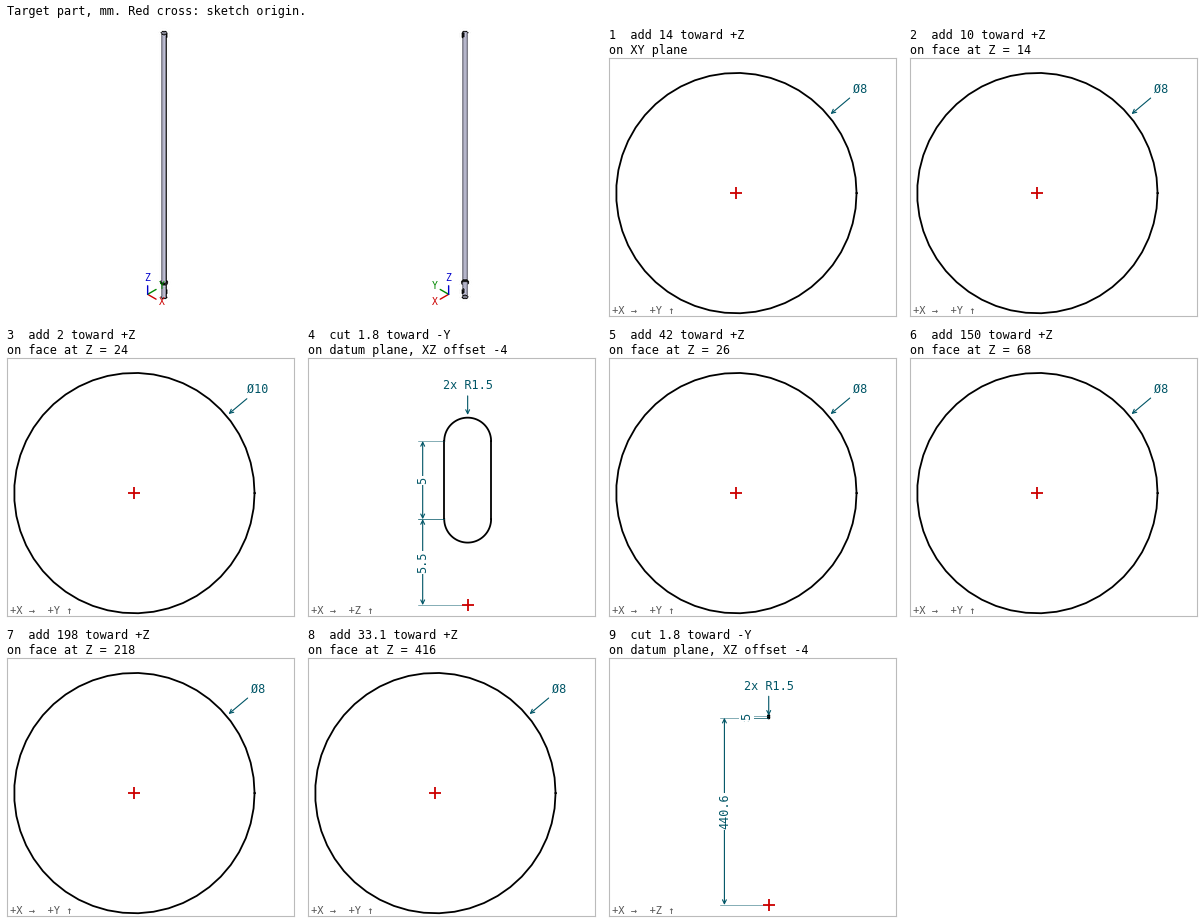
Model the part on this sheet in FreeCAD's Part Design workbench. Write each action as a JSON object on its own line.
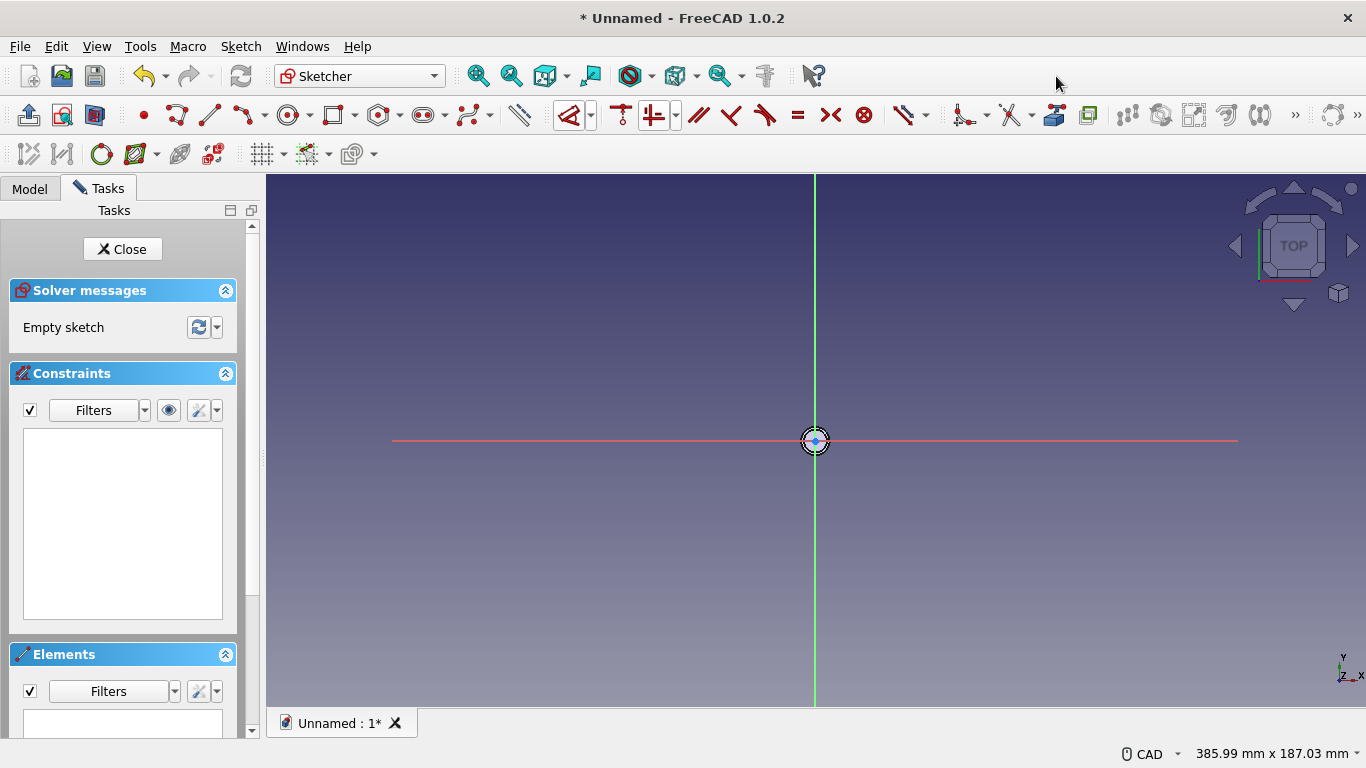
{"action": "scroll", "coordinate": [821, 441], "scroll_direction": "up", "scroll_amount": 13}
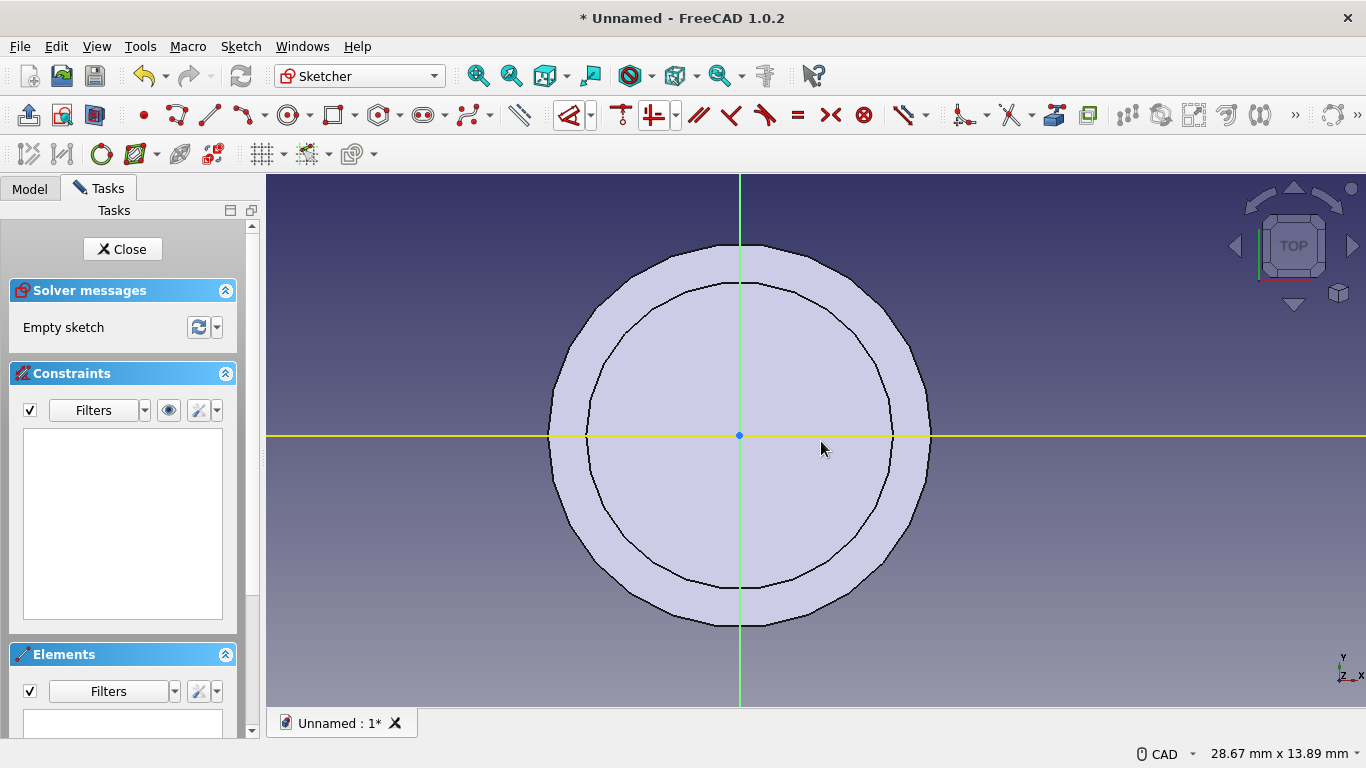
{"action": "left_click", "coordinate": [288, 116]}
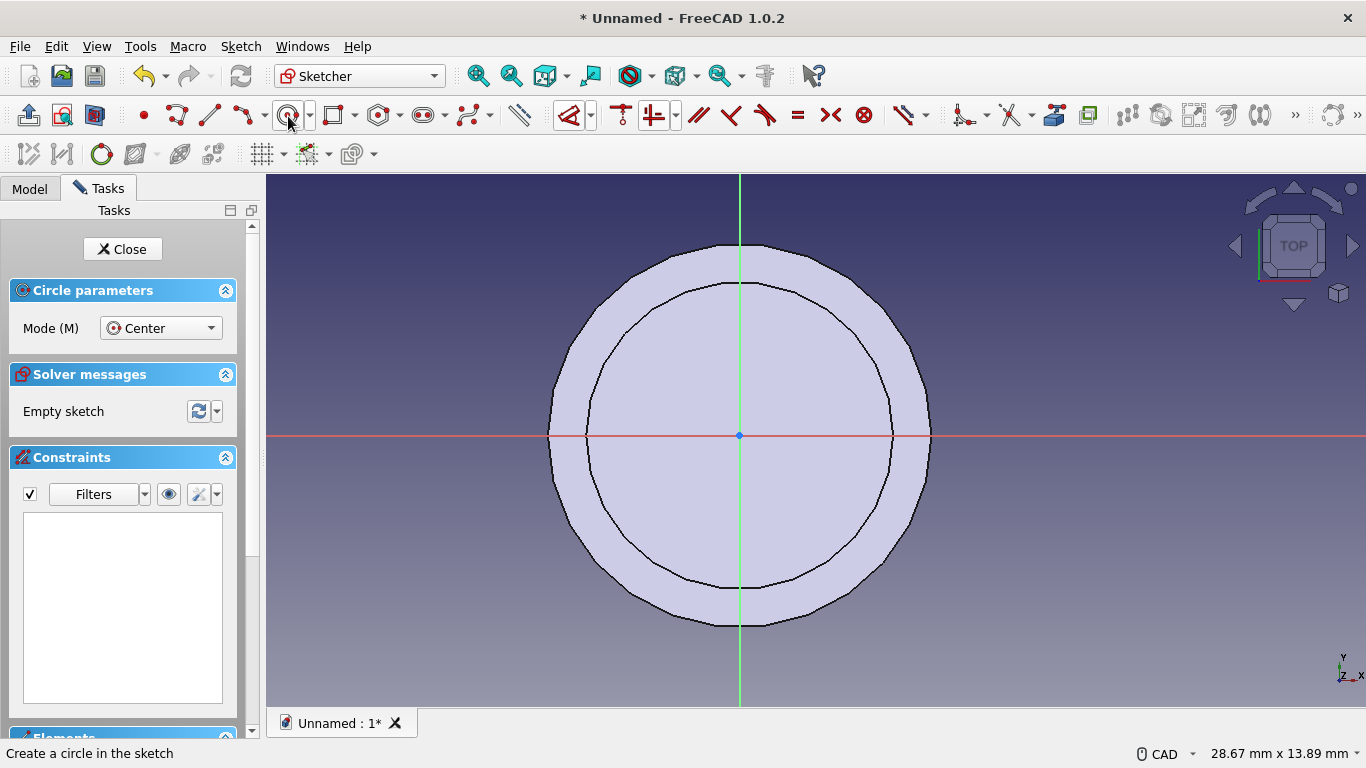
{"action": "left_click", "coordinate": [740, 436]}
{"action": "left_click", "coordinate": [848, 327]}
{"action": "key", "text": "Escape"}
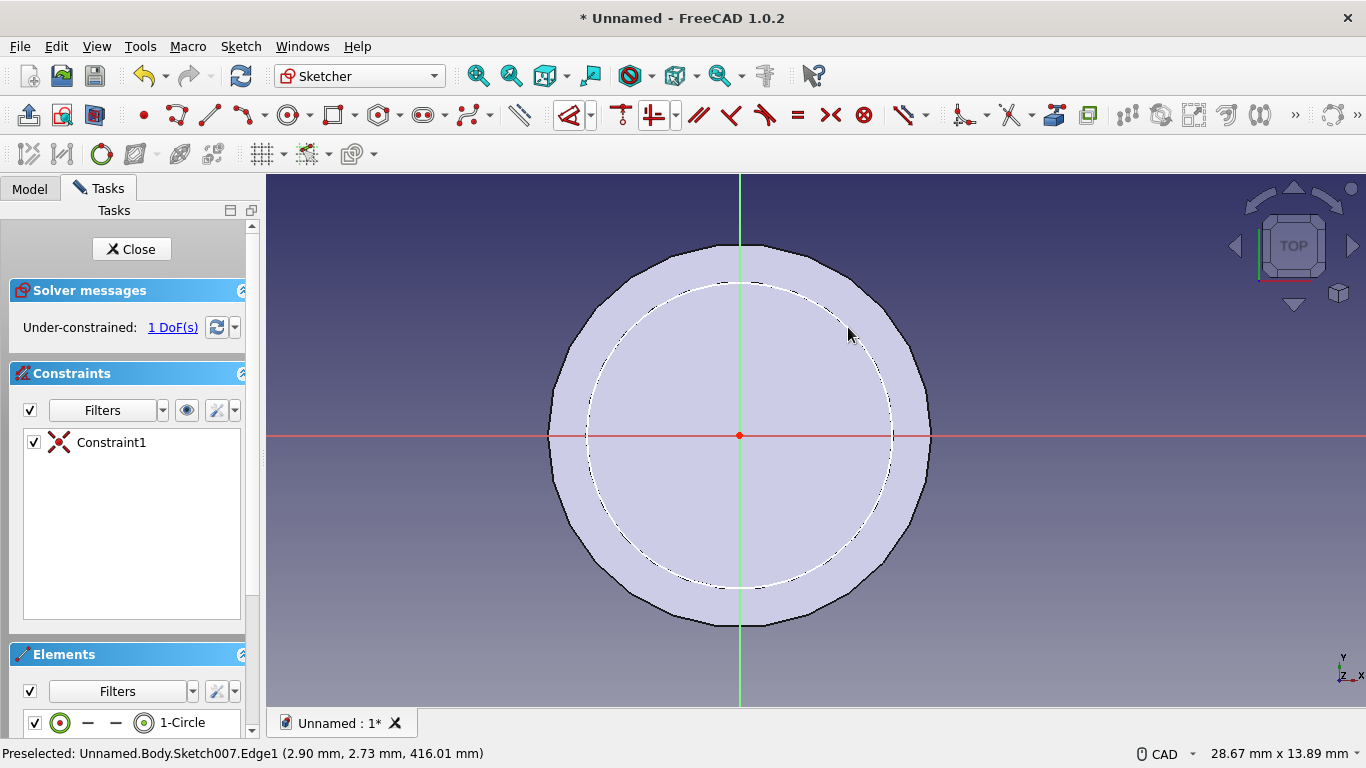
{"action": "left_click", "coordinate": [847, 327]}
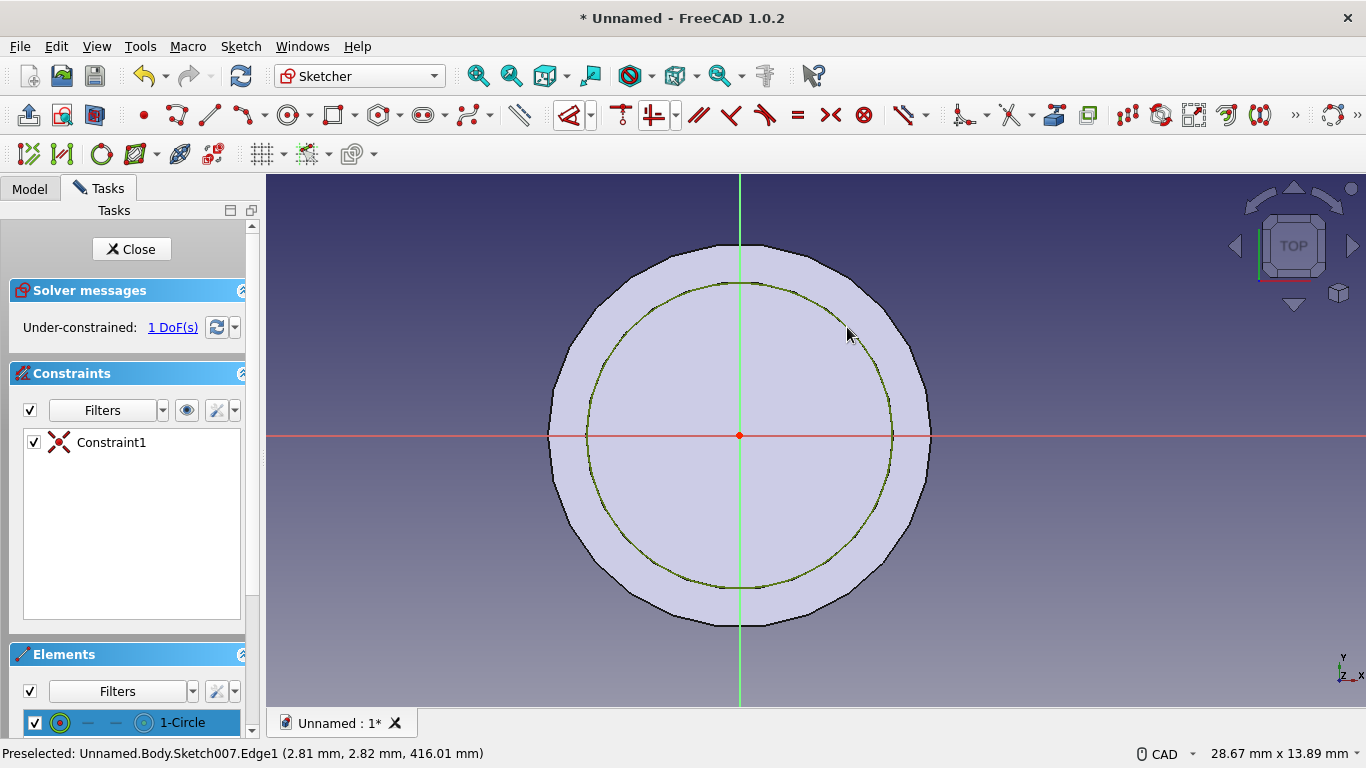
{"action": "key", "text": "k o"}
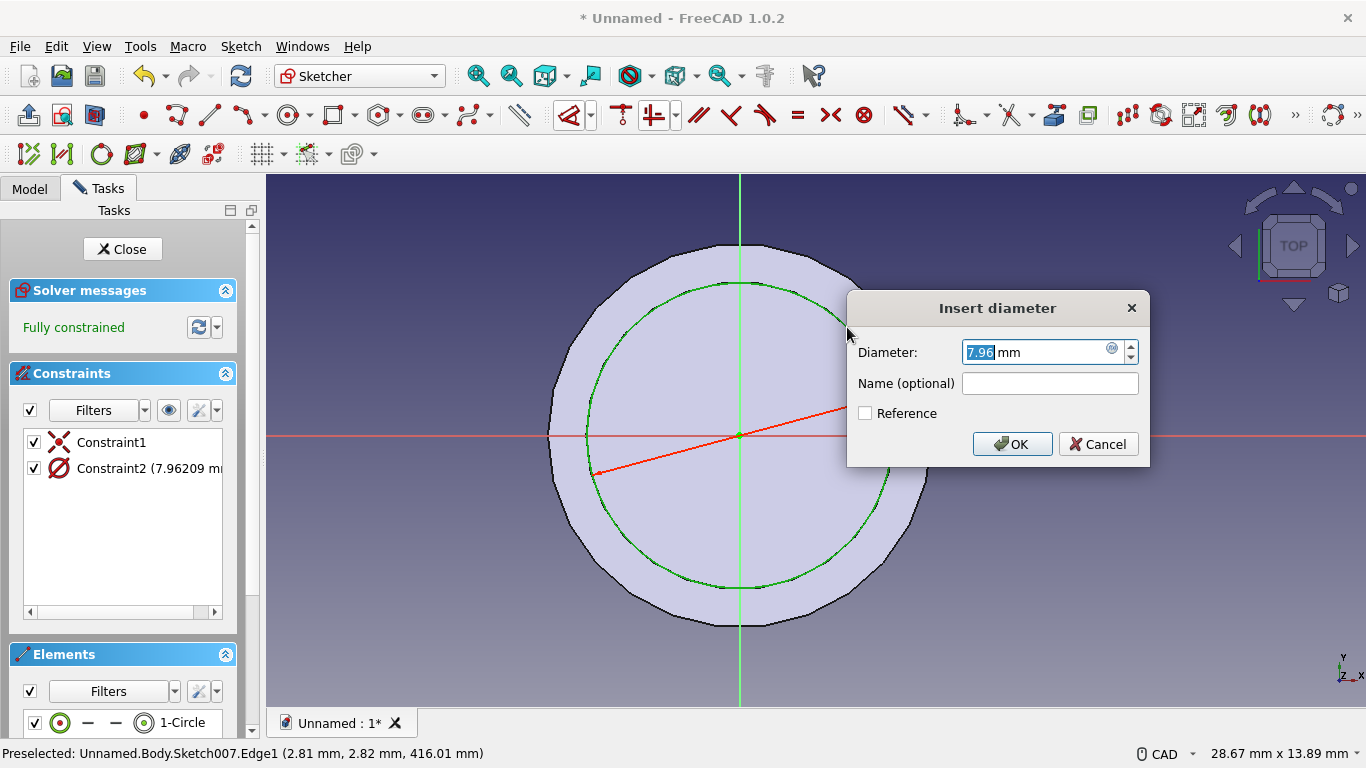
{"action": "type", "text": "8"}
{"action": "key", "text": "Return"}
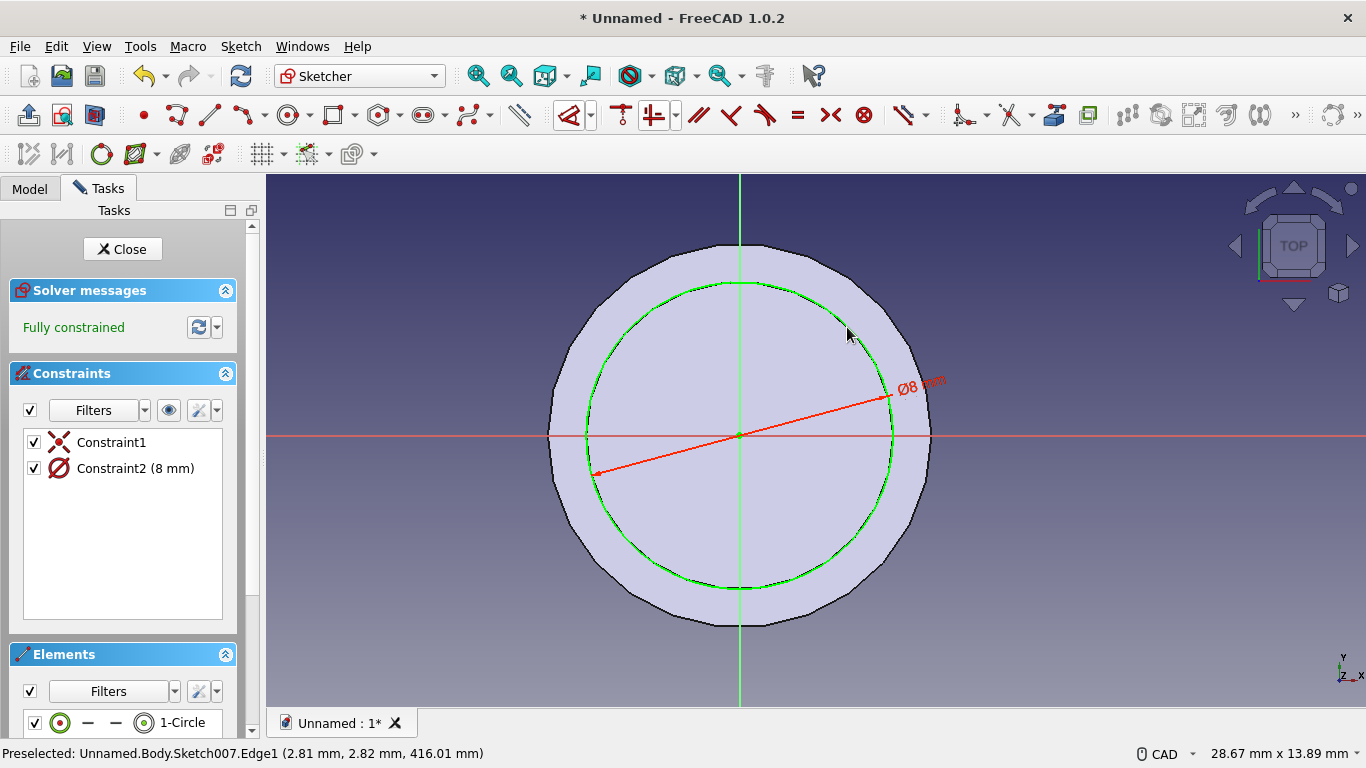
{"action": "left_click", "coordinate": [123, 249]}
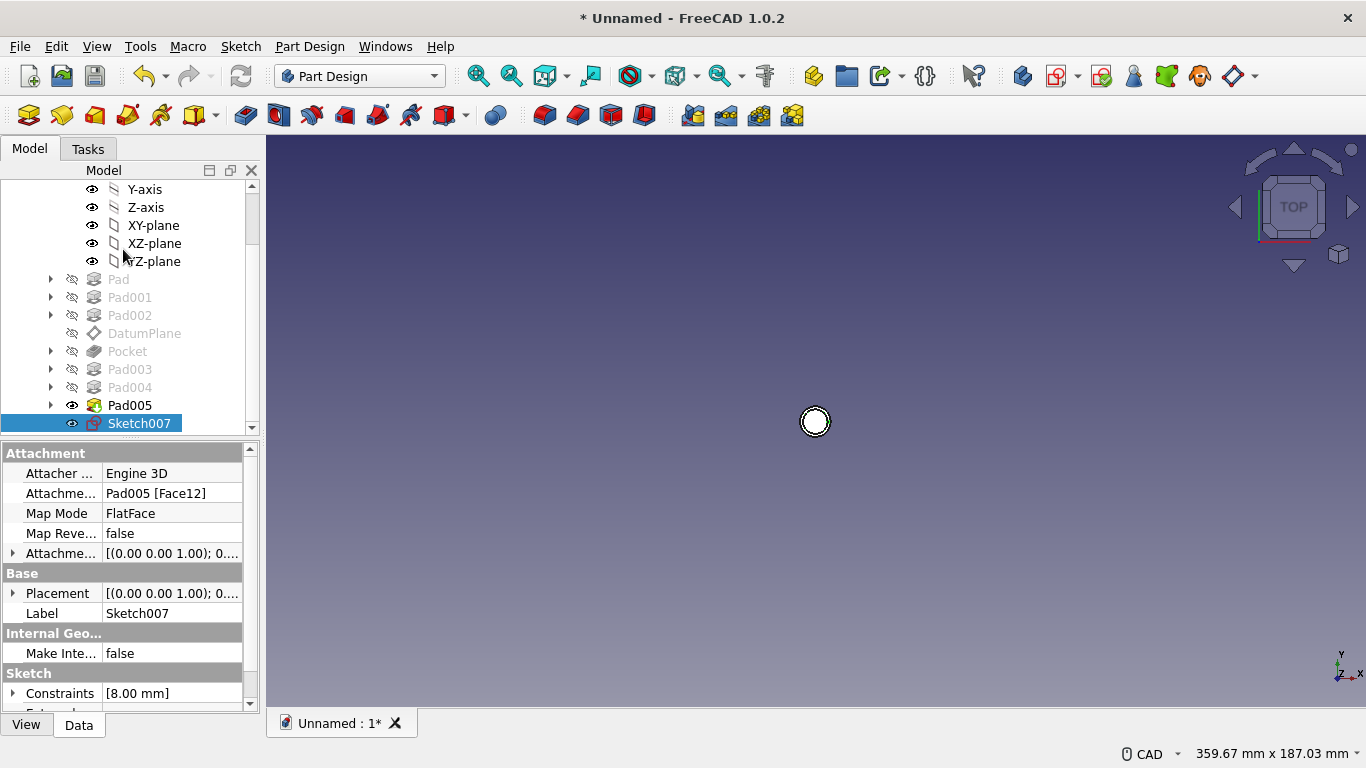
{"action": "left_click", "coordinate": [29, 116]}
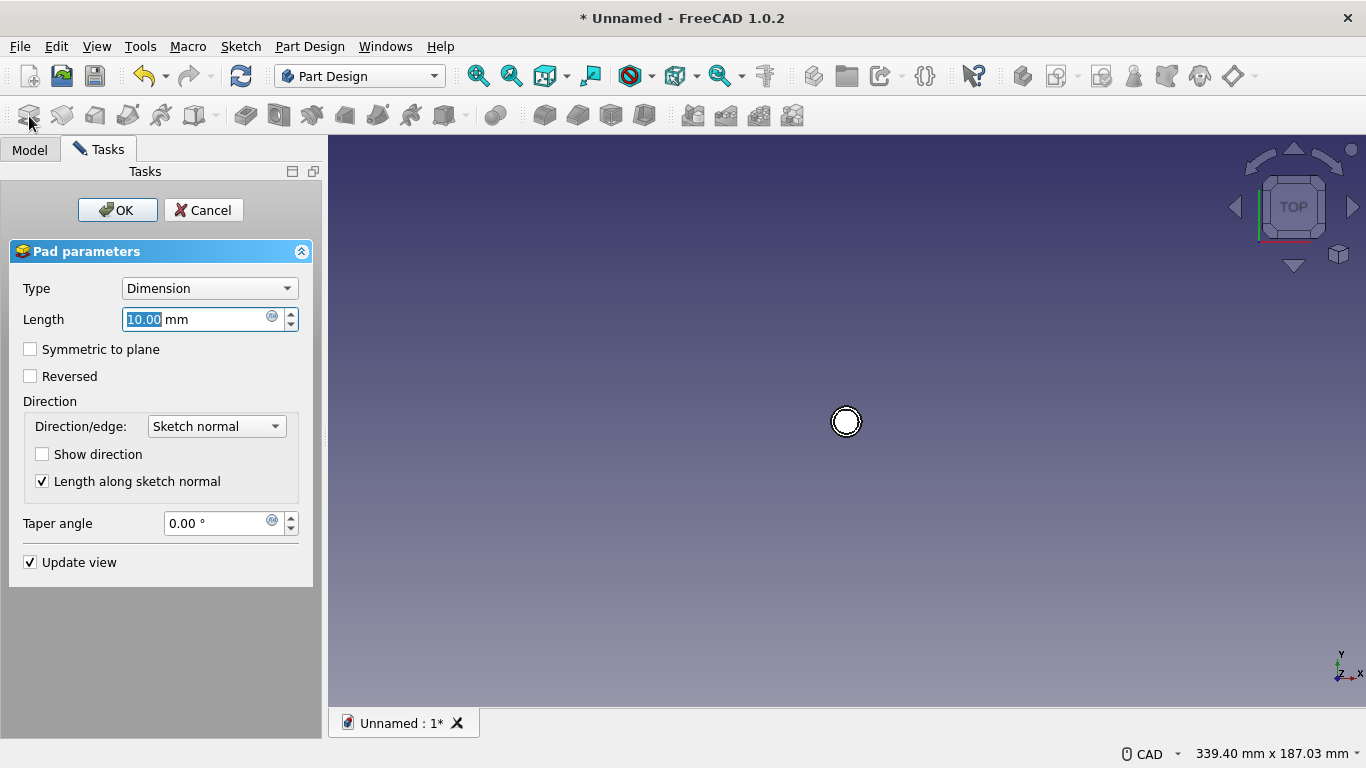
{"action": "type", "text": "33.1"}
{"action": "key", "text": "Tab"}